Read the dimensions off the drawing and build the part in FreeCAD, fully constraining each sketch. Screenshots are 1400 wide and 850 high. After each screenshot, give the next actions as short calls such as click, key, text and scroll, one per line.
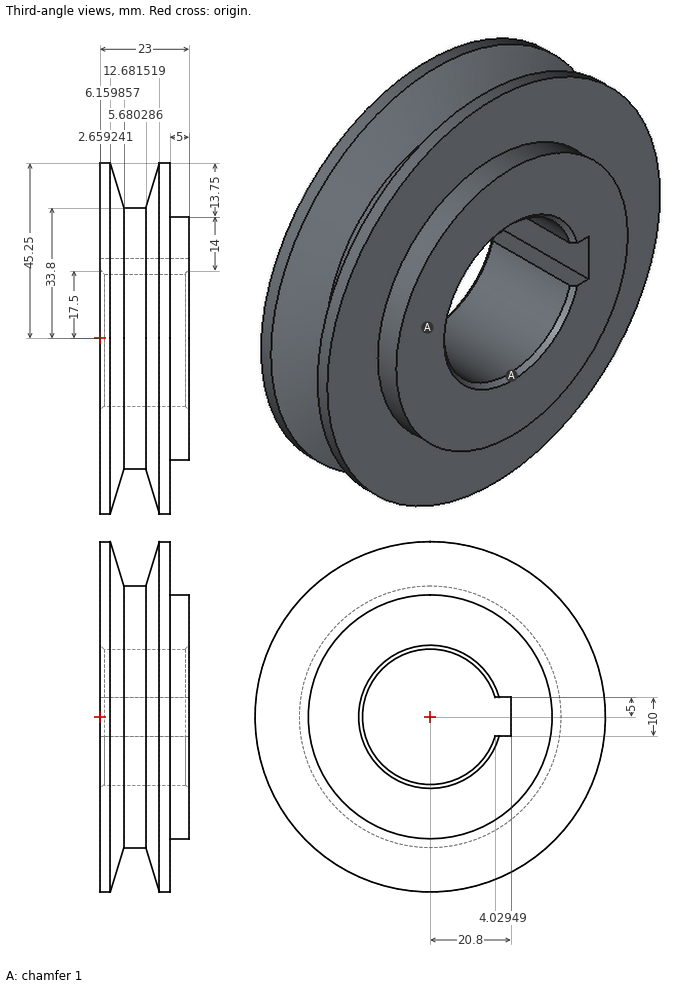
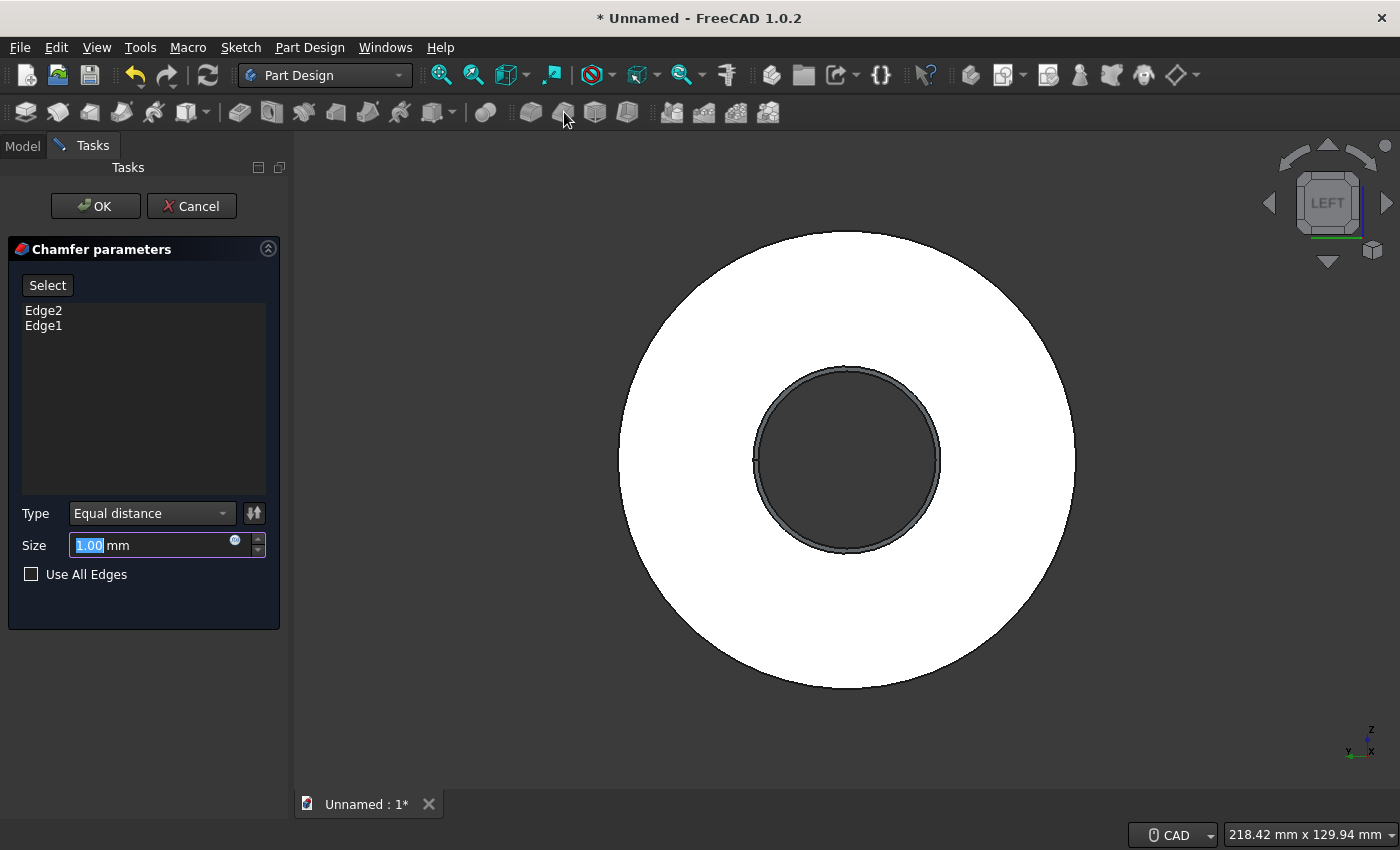
text(1)
key(Tab)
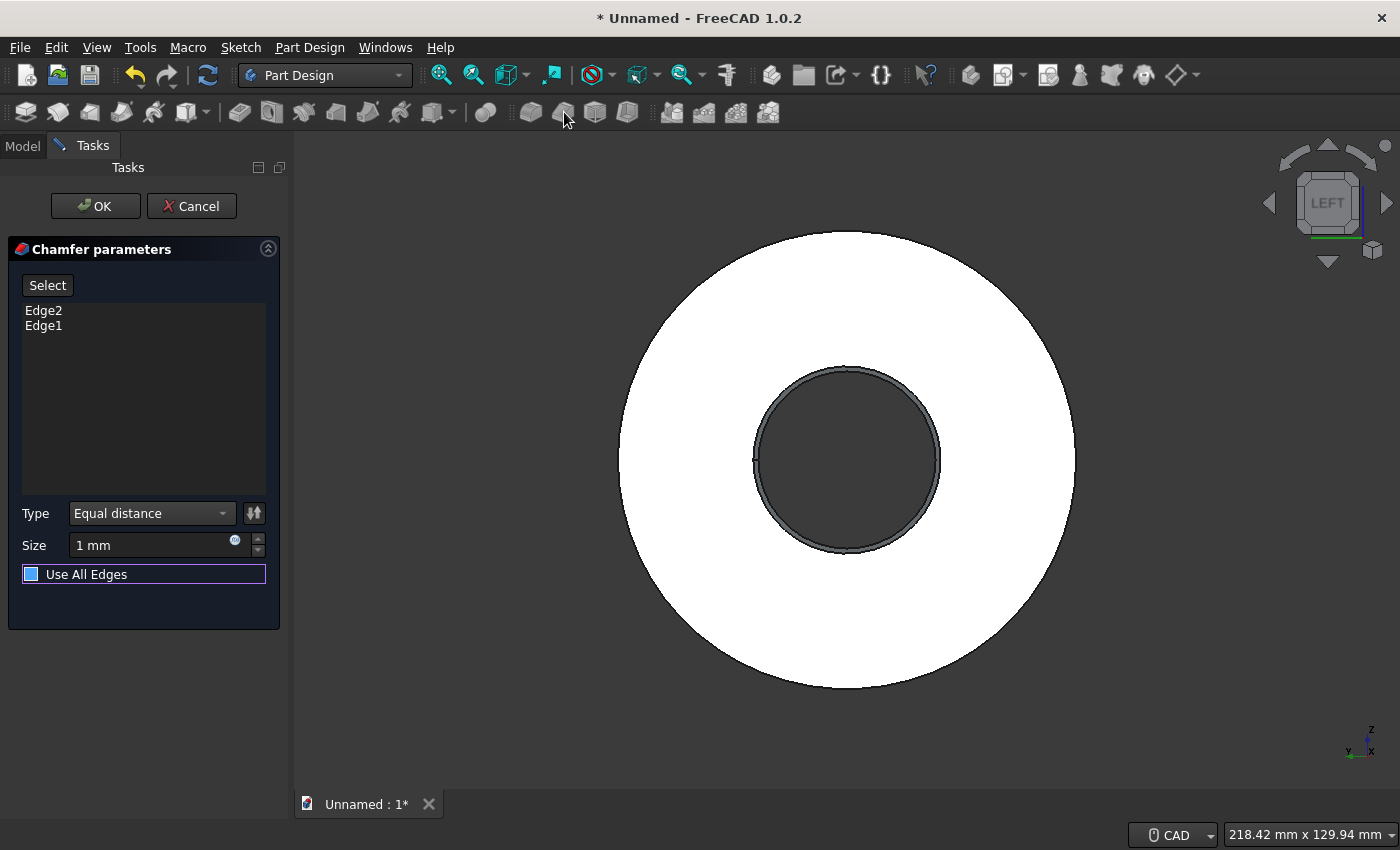
click(96, 206)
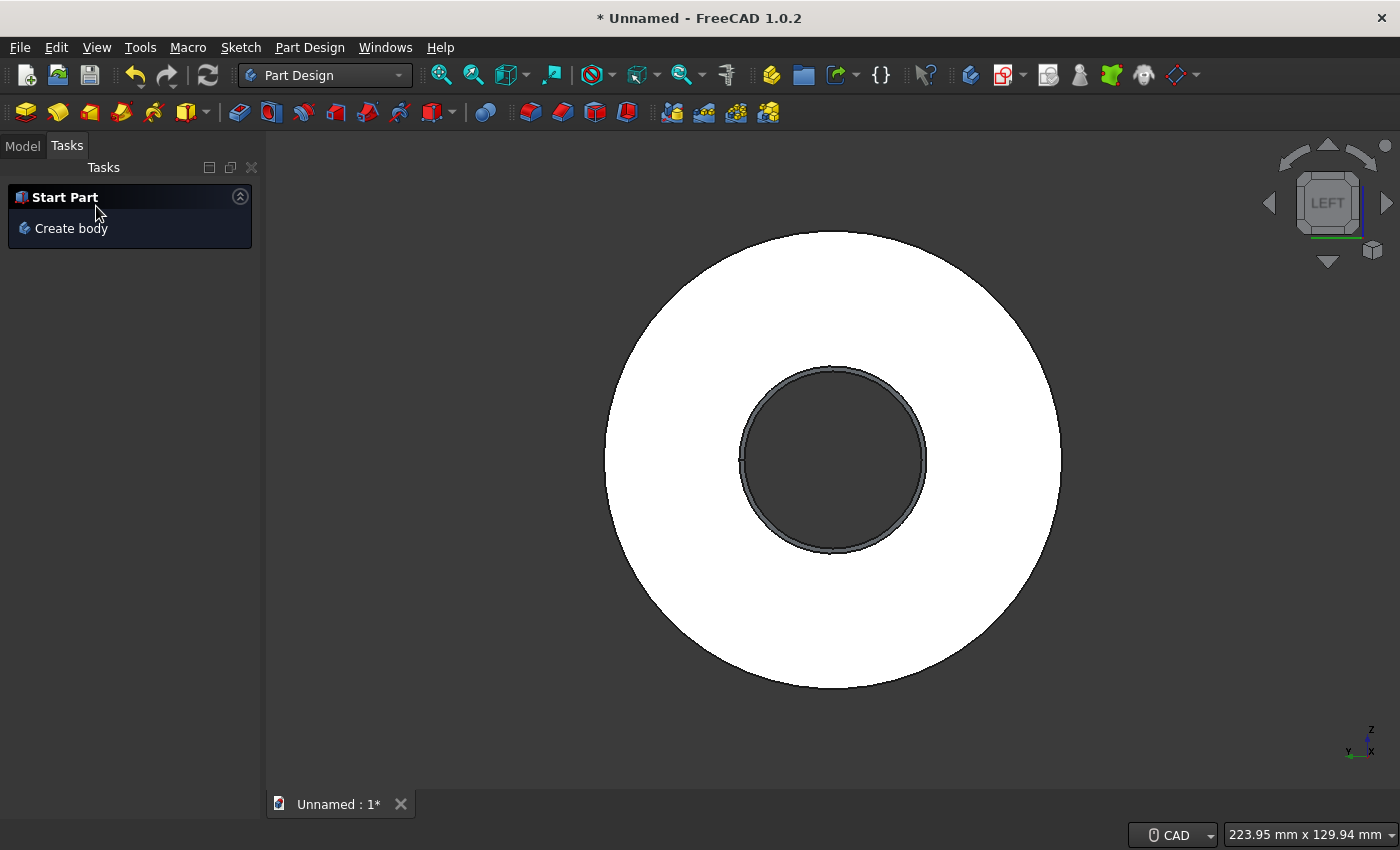
click(1004, 76)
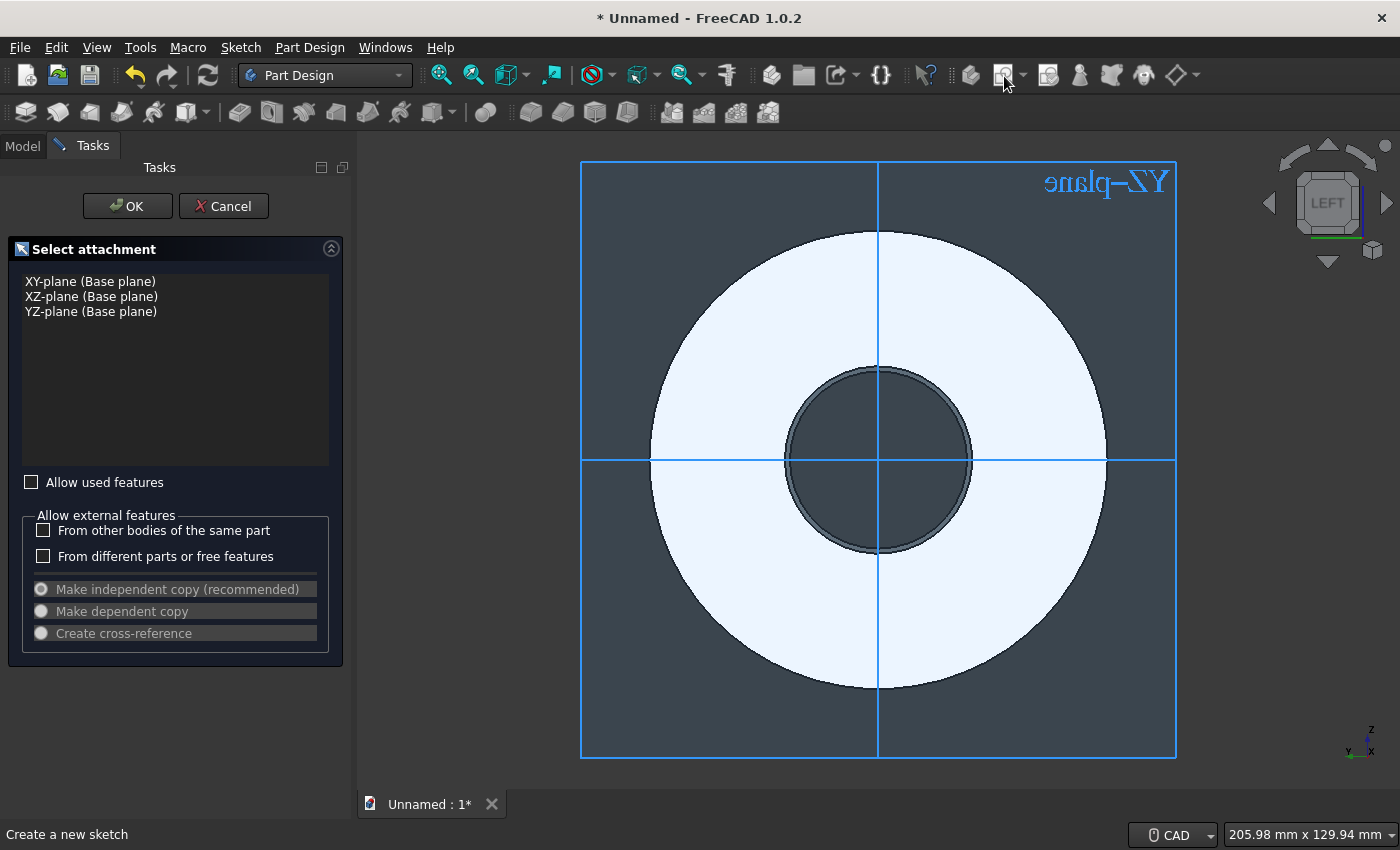
click(82, 312)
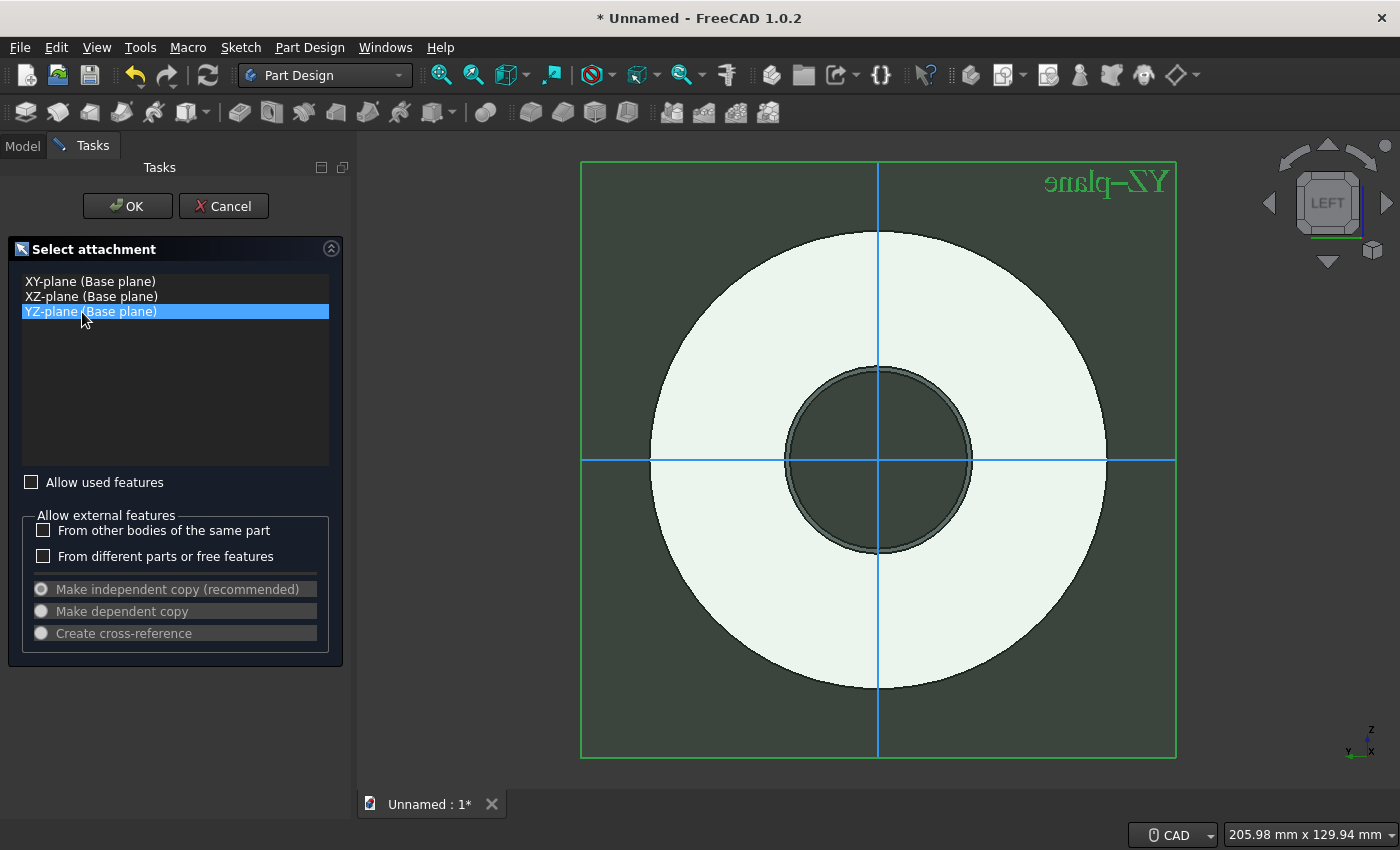
click(128, 206)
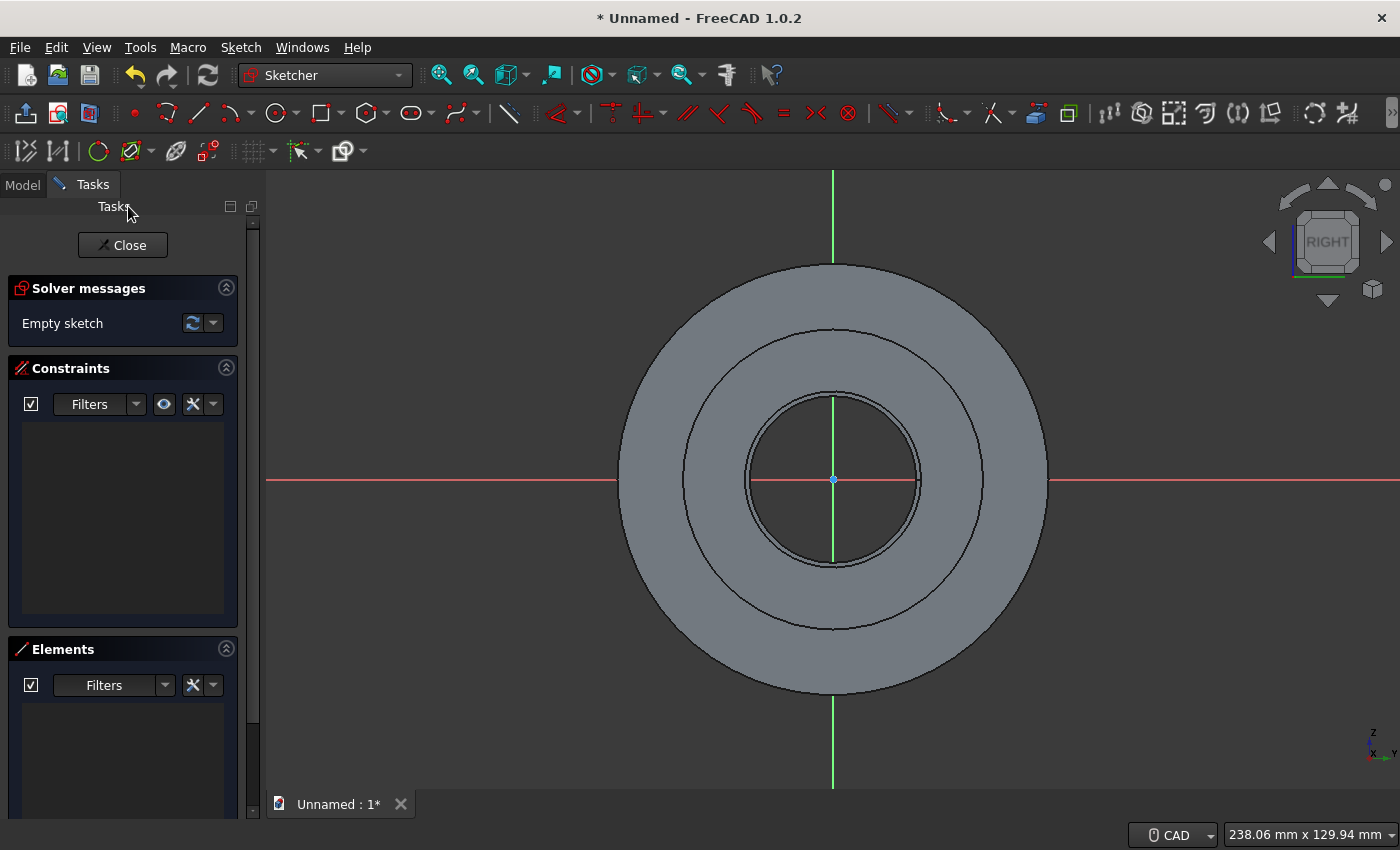
key(q)
key(s)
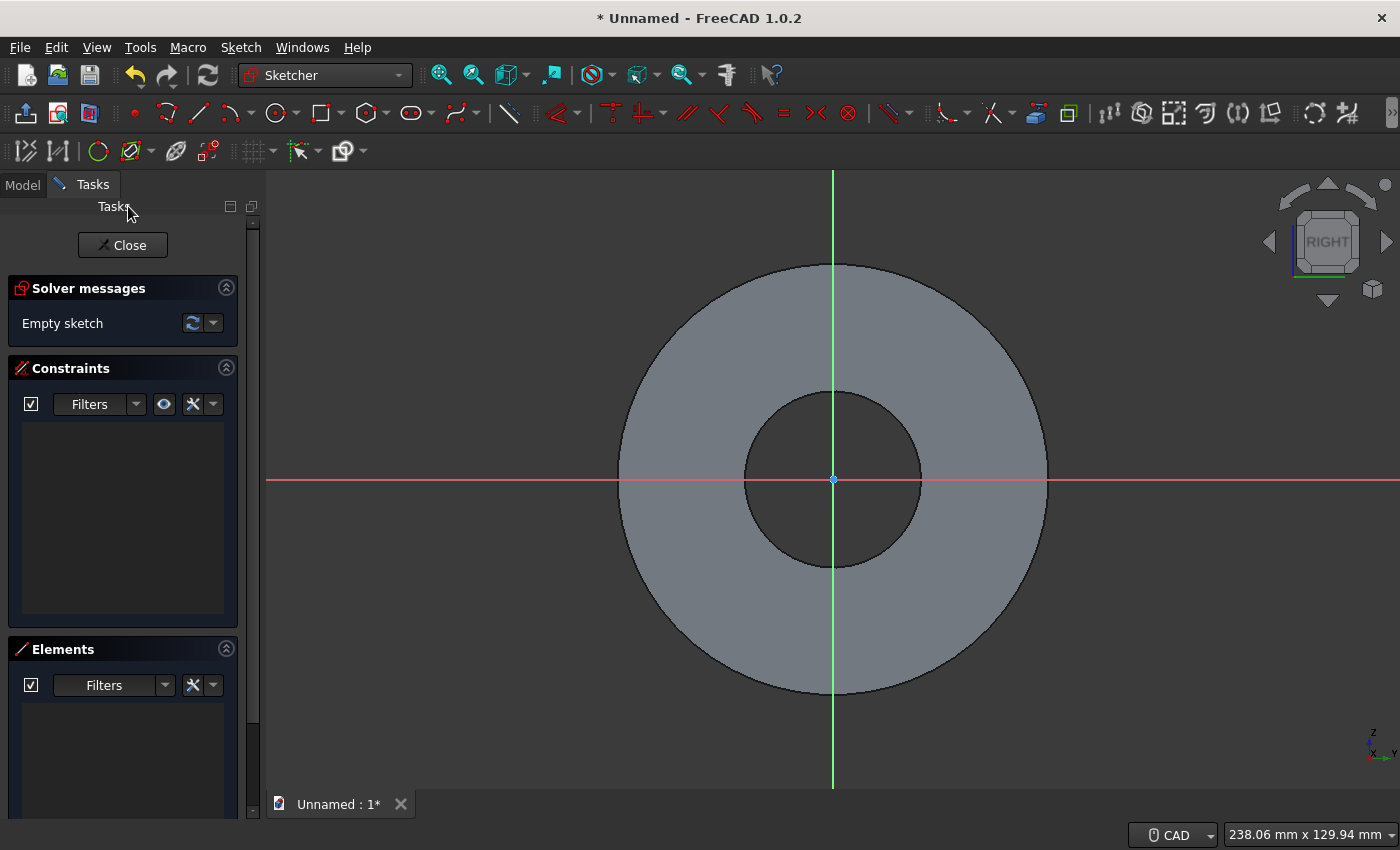
scroll(901, 479, up, 10)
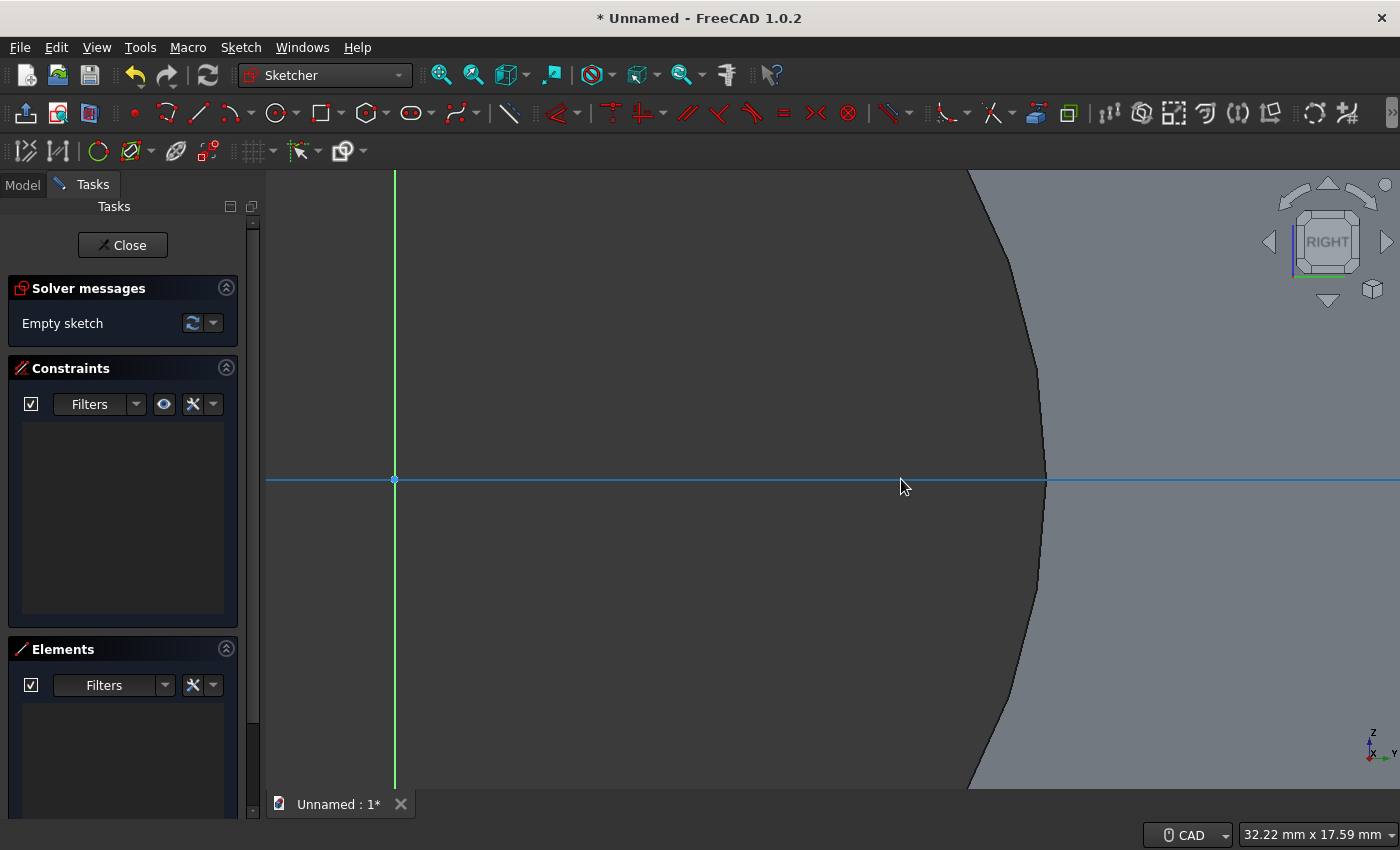
click(322, 114)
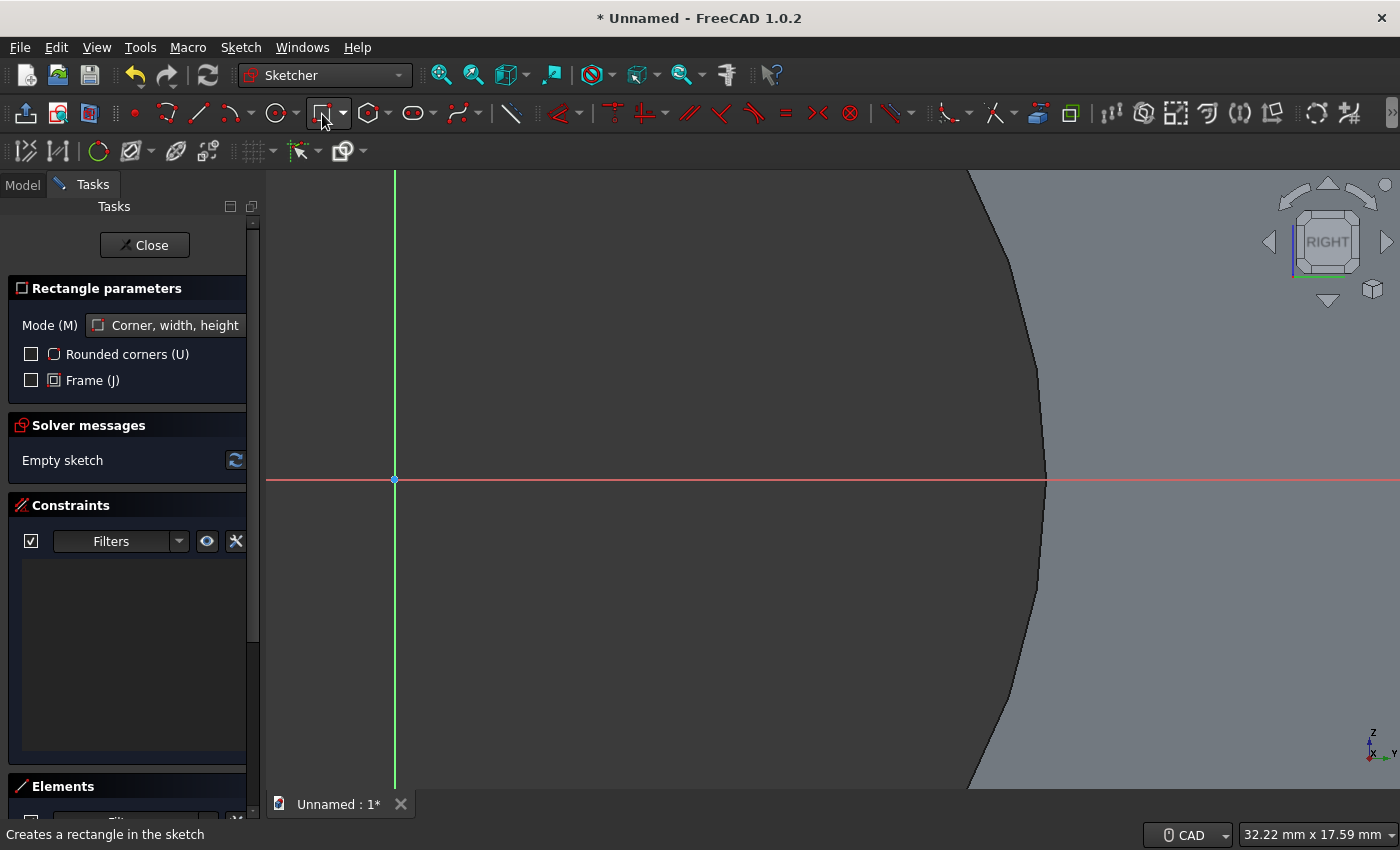
click(985, 304)
move(1127, 655)